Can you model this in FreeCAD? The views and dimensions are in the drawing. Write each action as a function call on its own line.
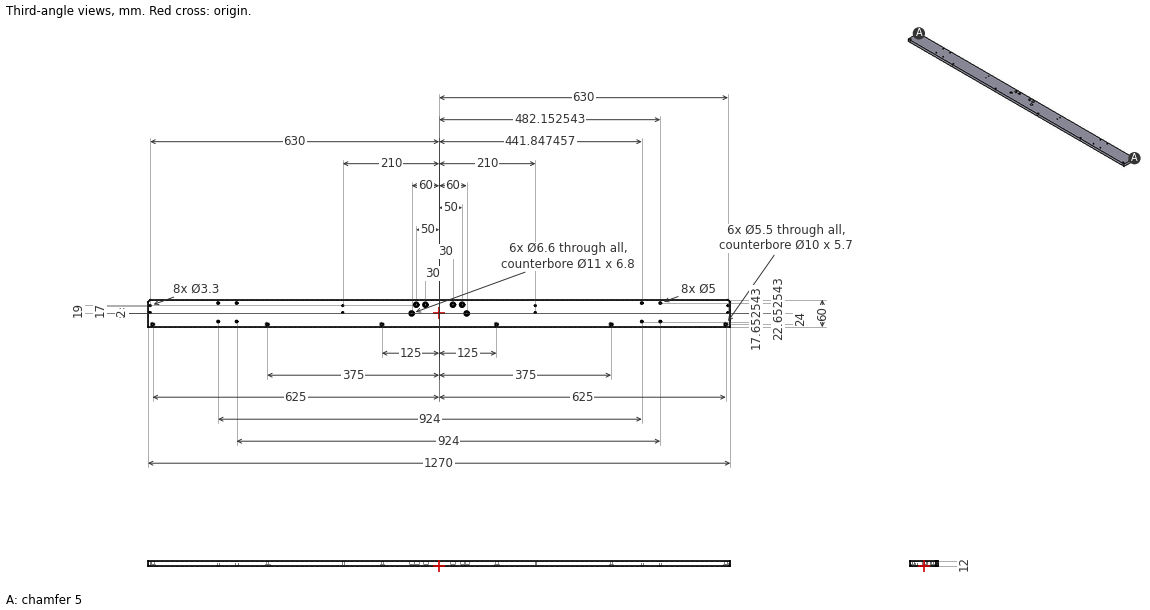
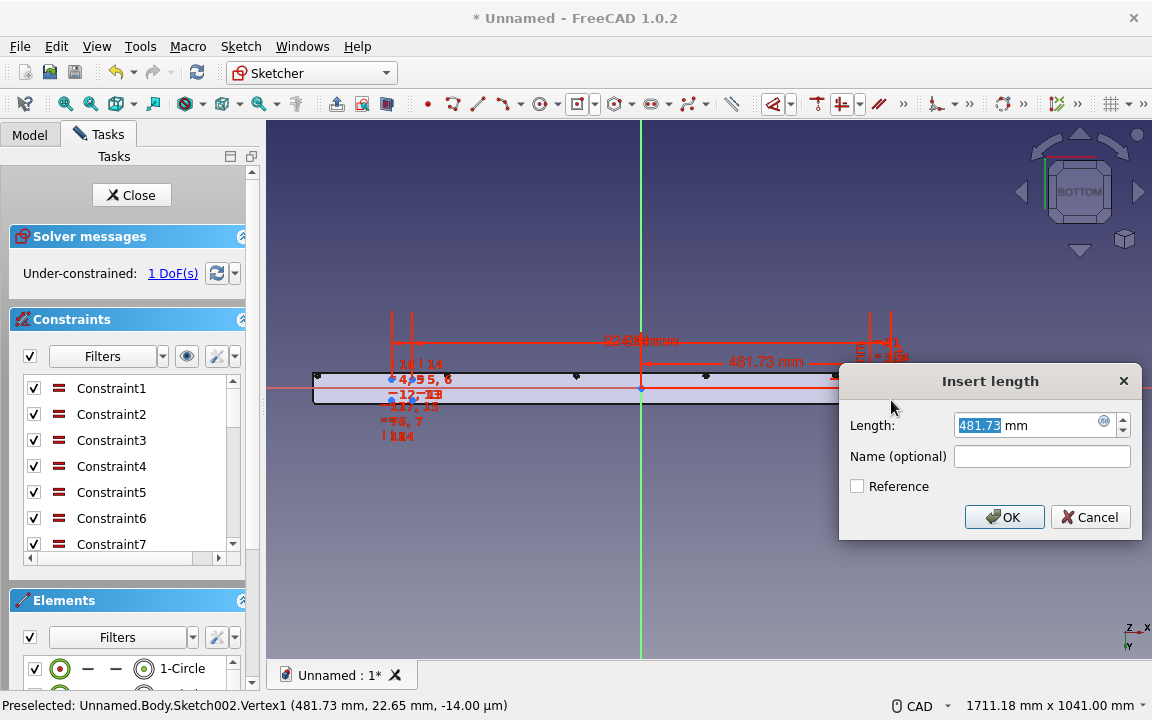
text(482.152543)
key(Return)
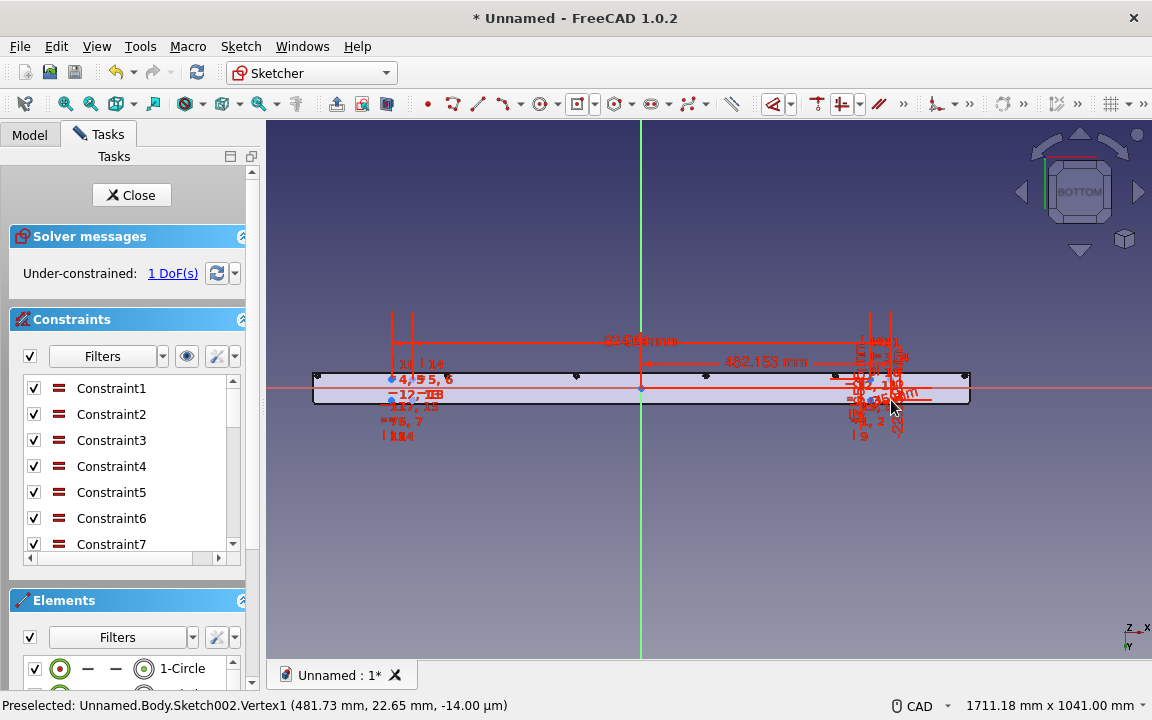
click(870, 400)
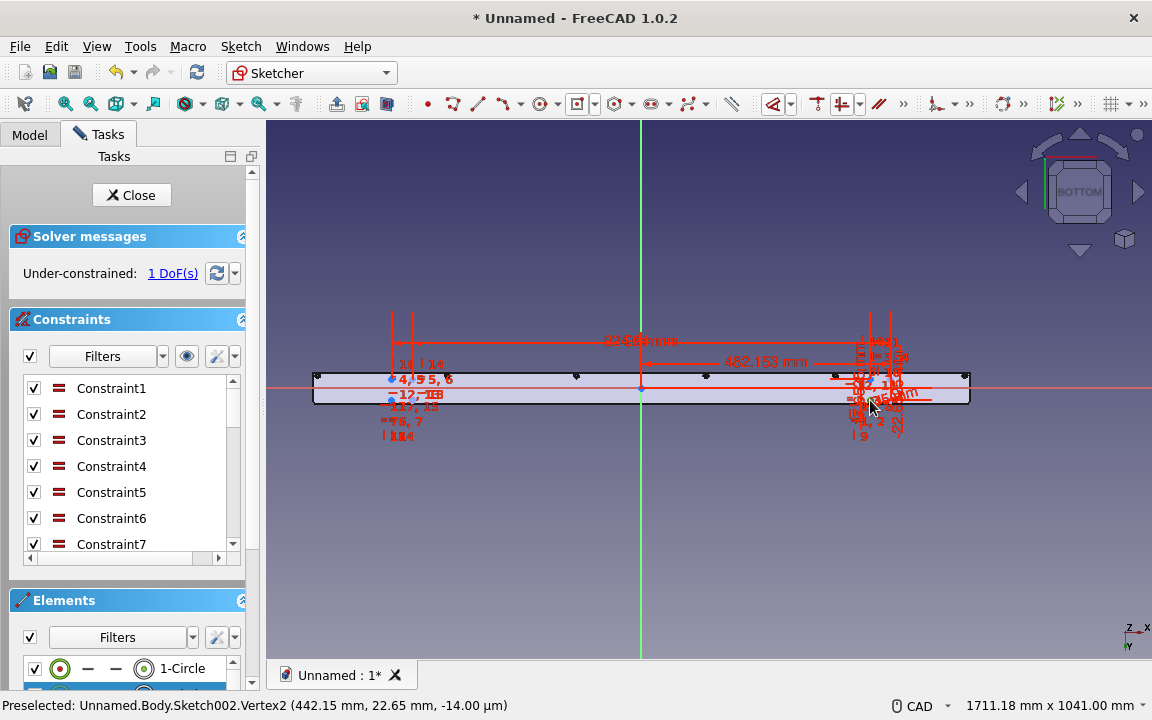
click(790, 104)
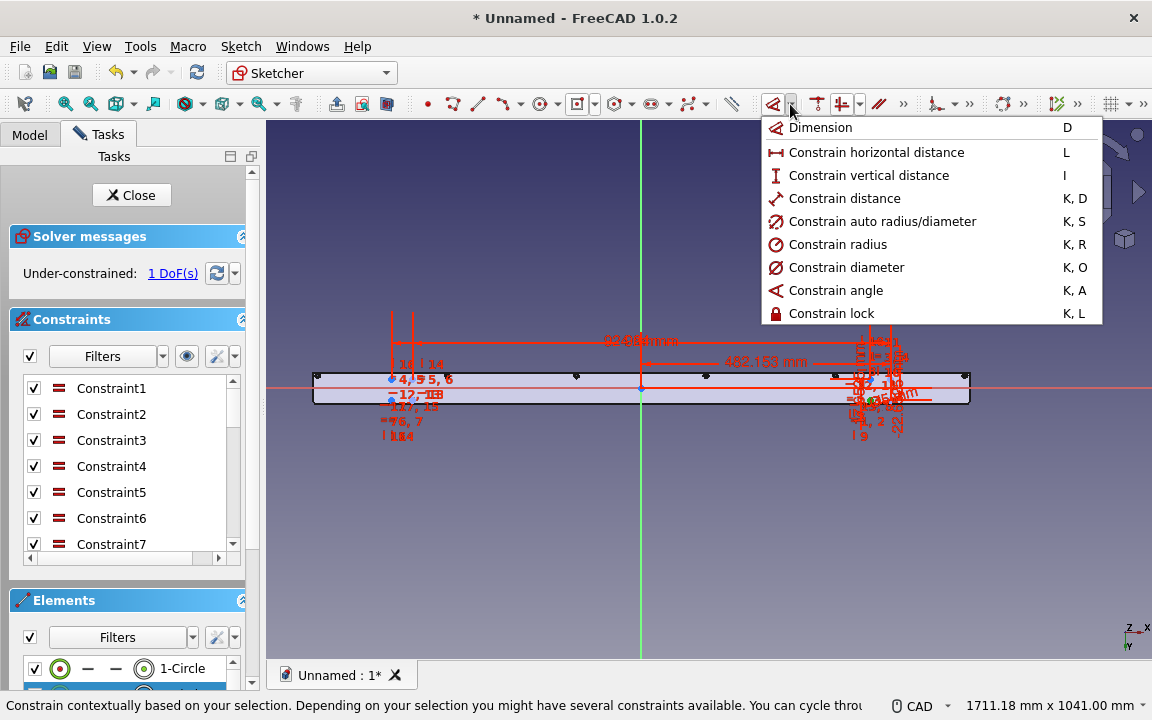
click(932, 152)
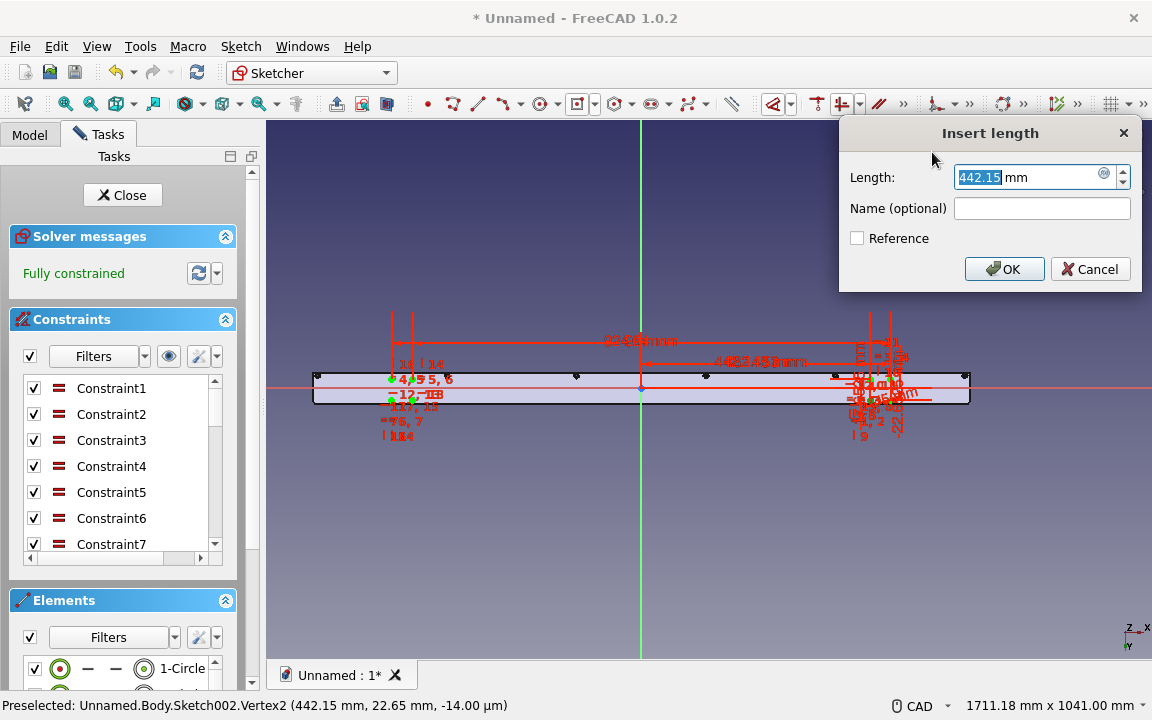
text(441.847457)
key(Return)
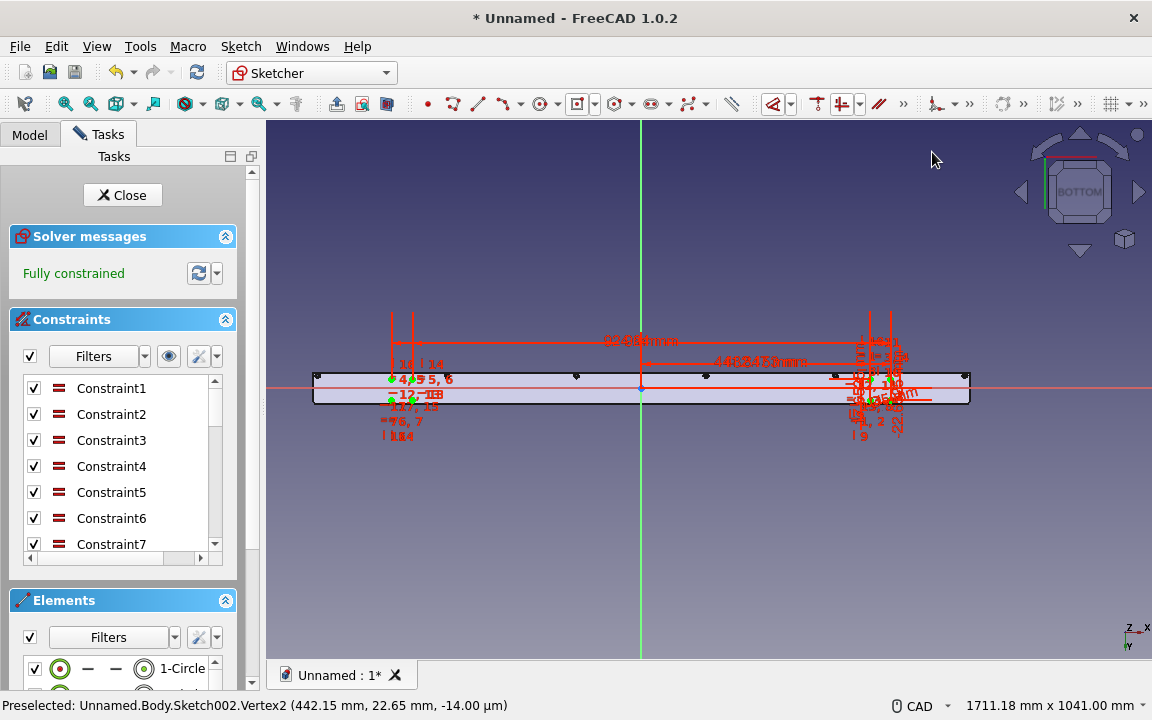
click(123, 195)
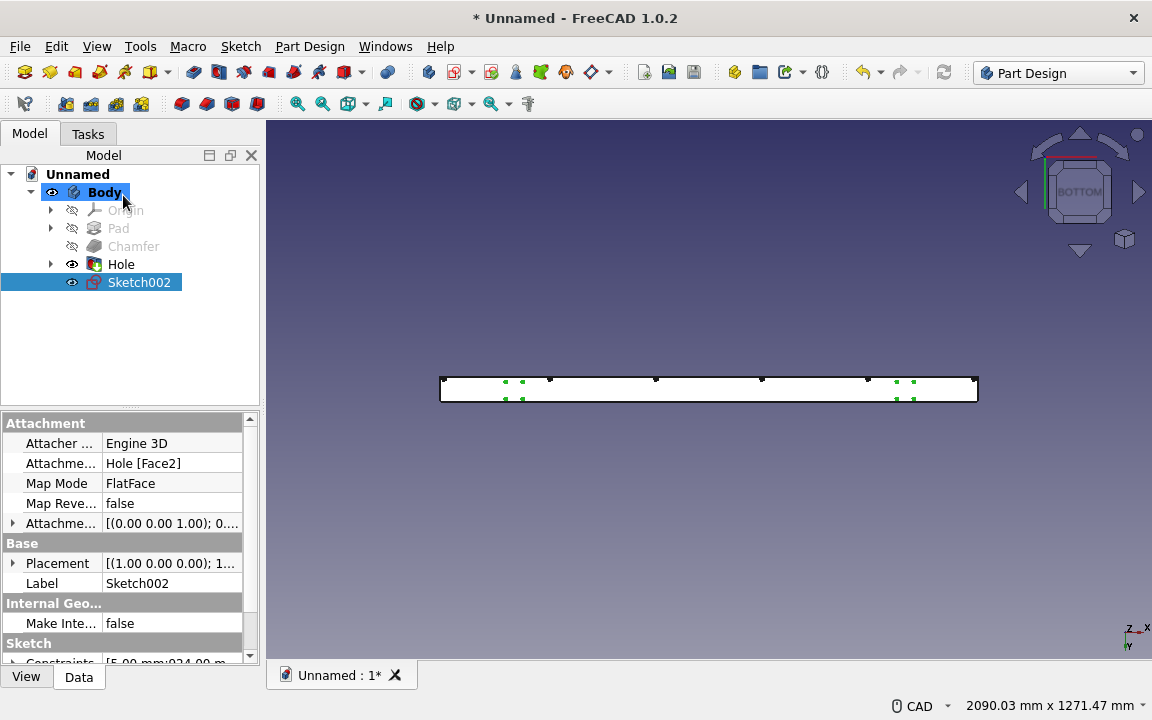
click(194, 72)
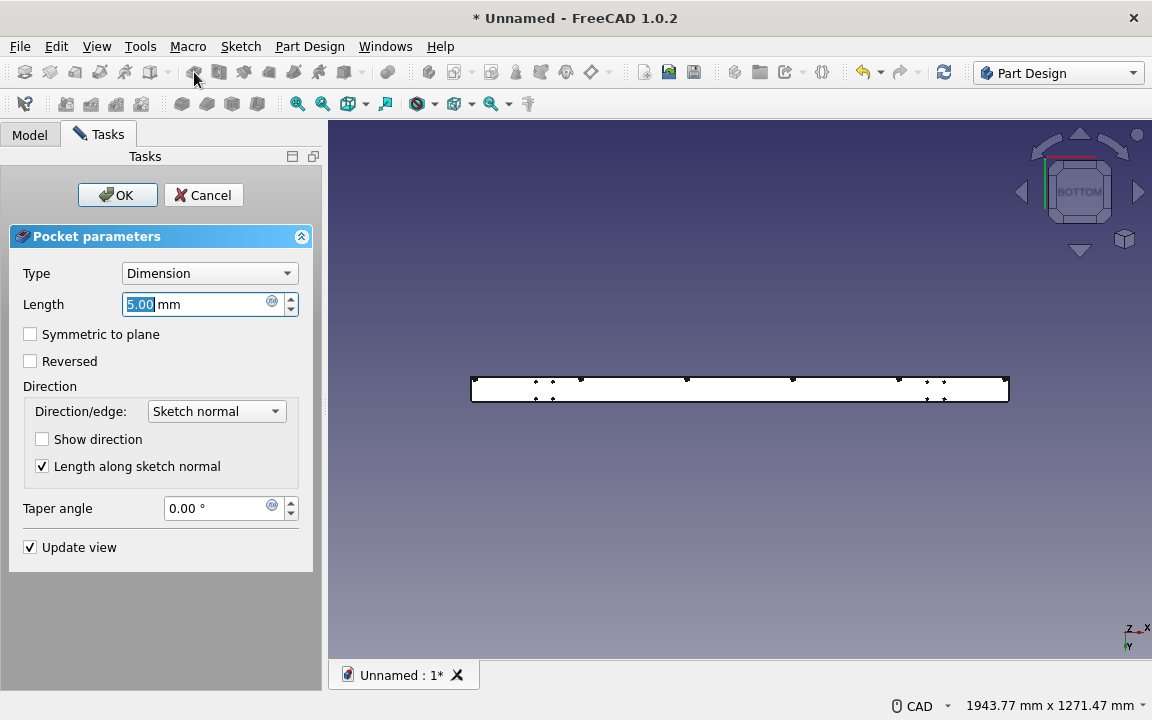
click(210, 274)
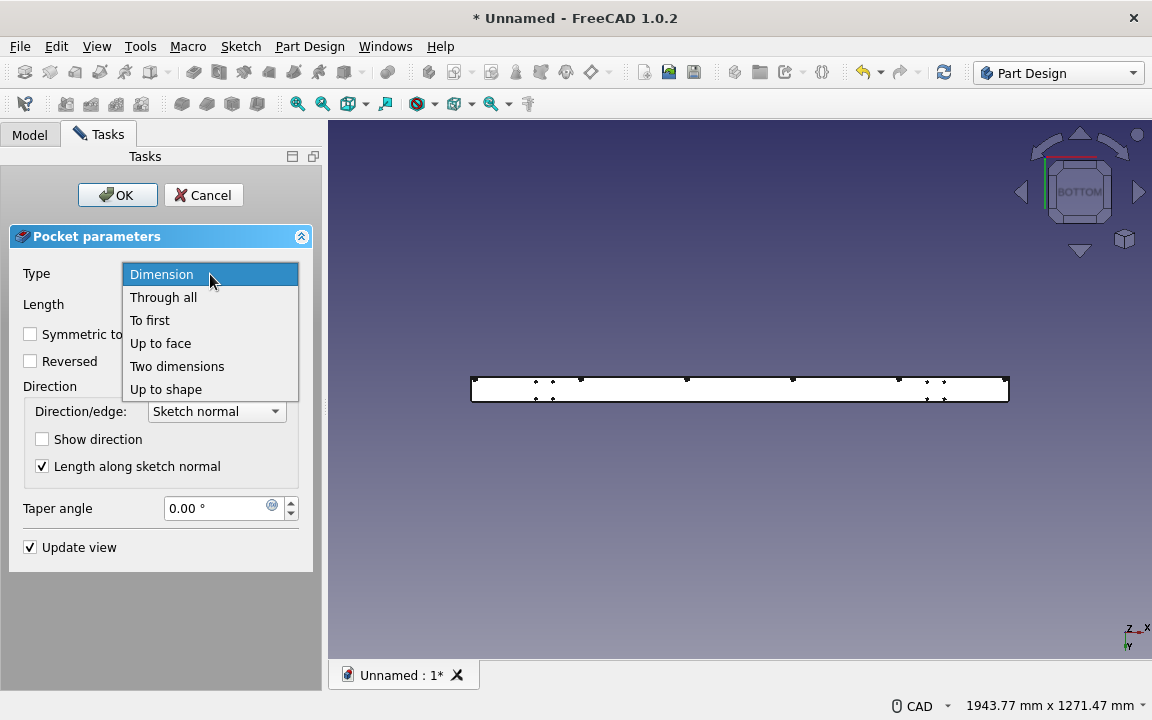
click(208, 298)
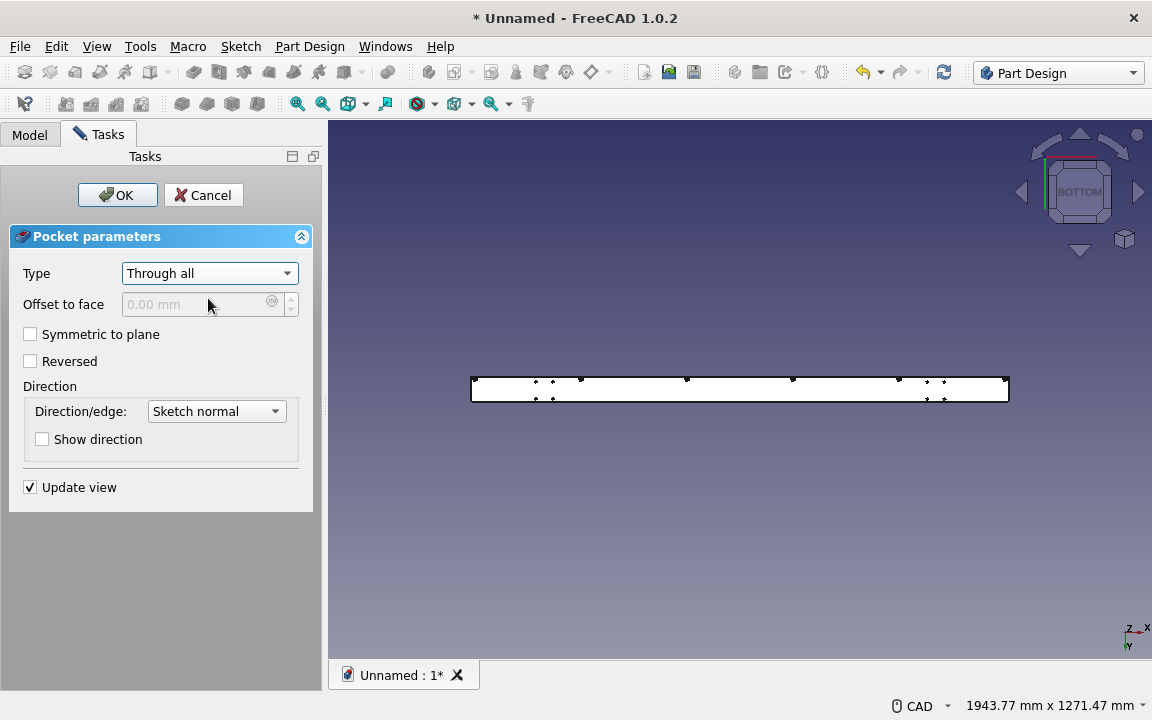
click(118, 195)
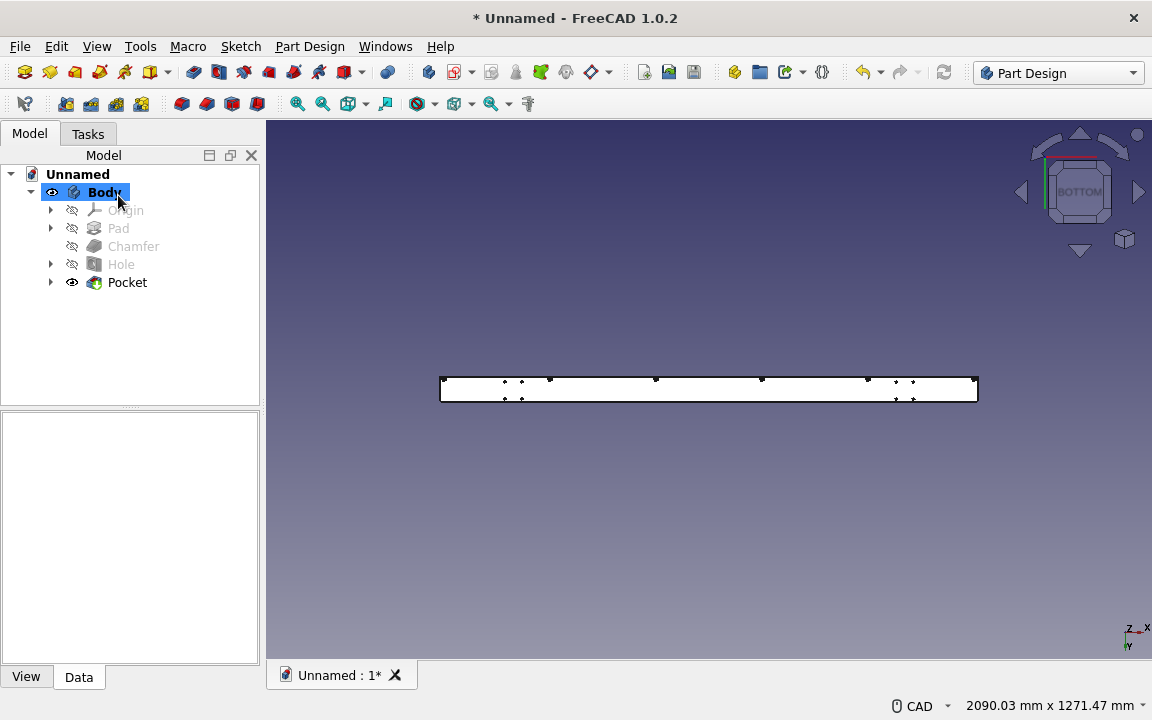
key(0)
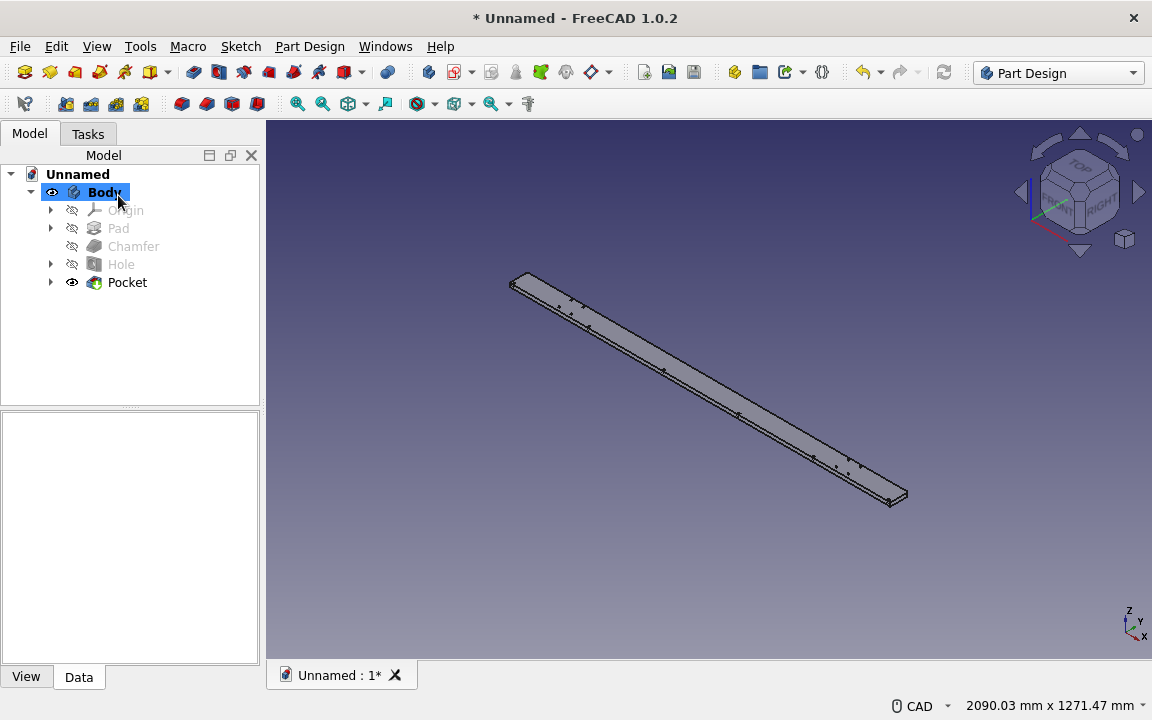
click(298, 104)